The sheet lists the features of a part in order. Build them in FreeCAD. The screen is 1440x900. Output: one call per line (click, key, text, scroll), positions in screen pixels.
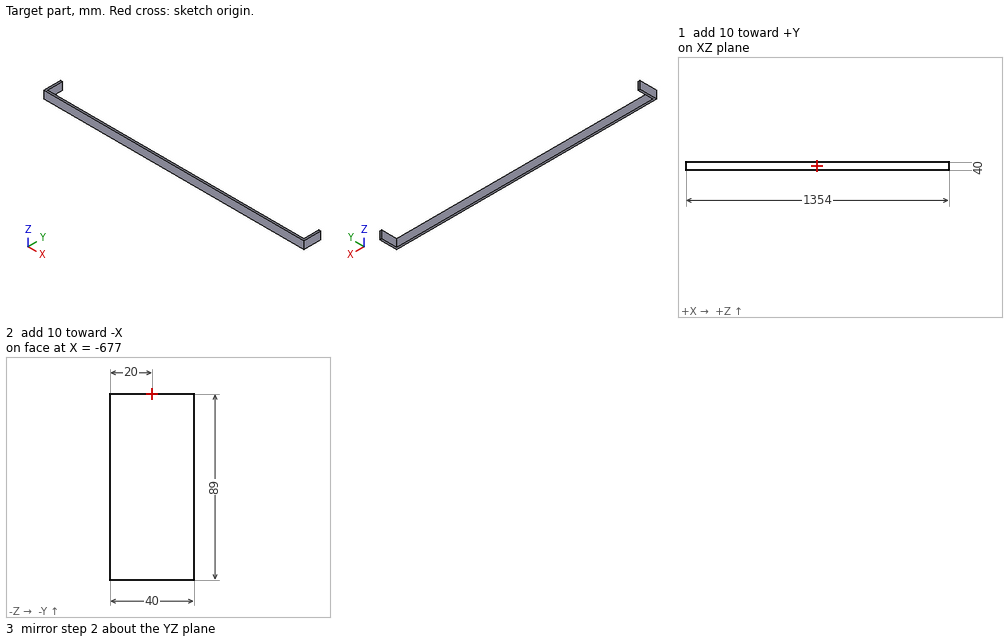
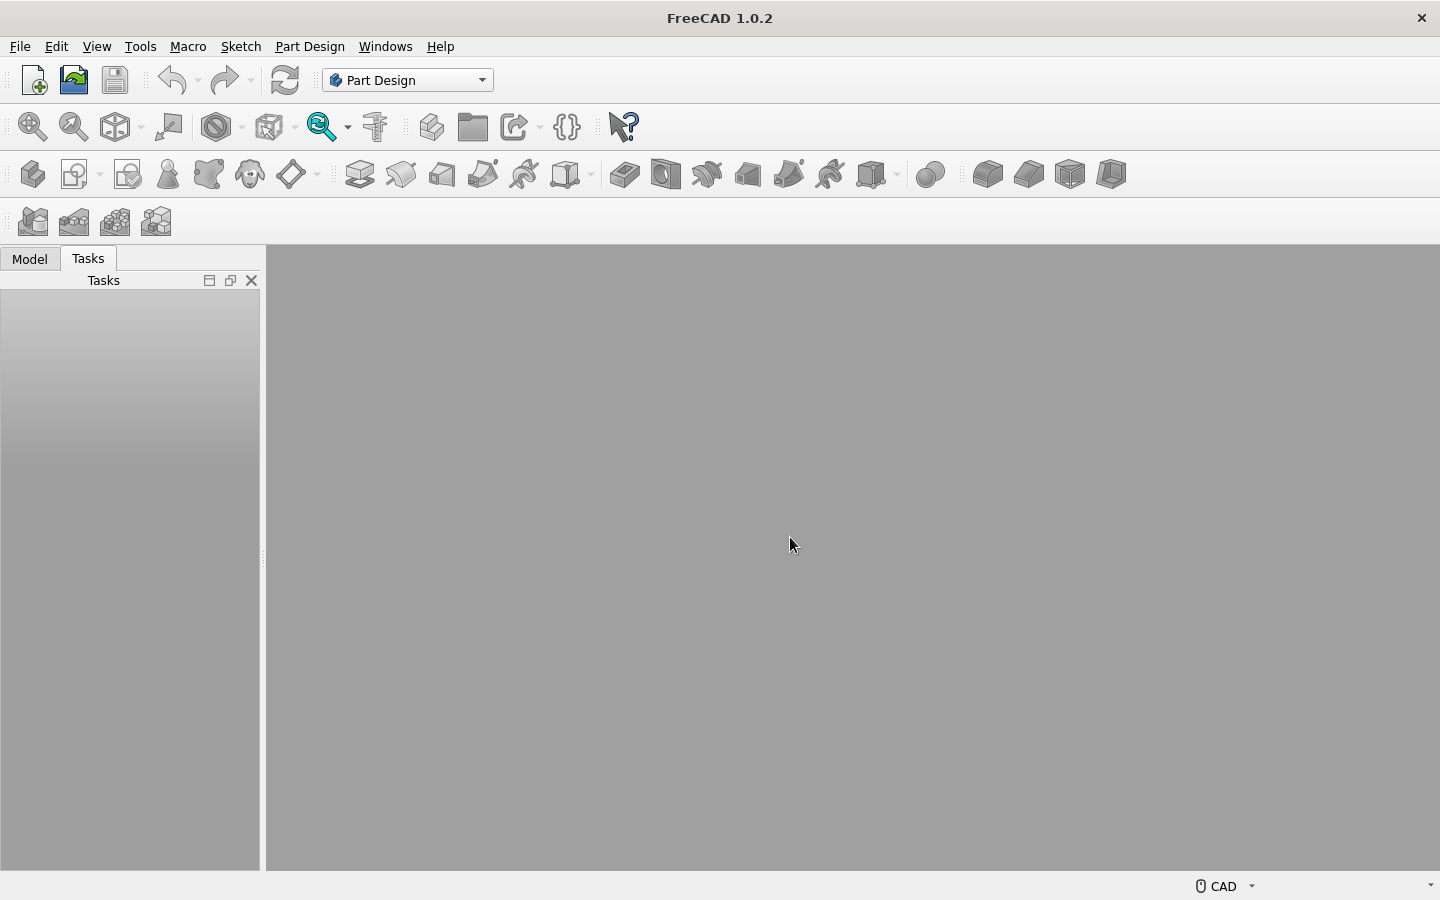
click(33, 80)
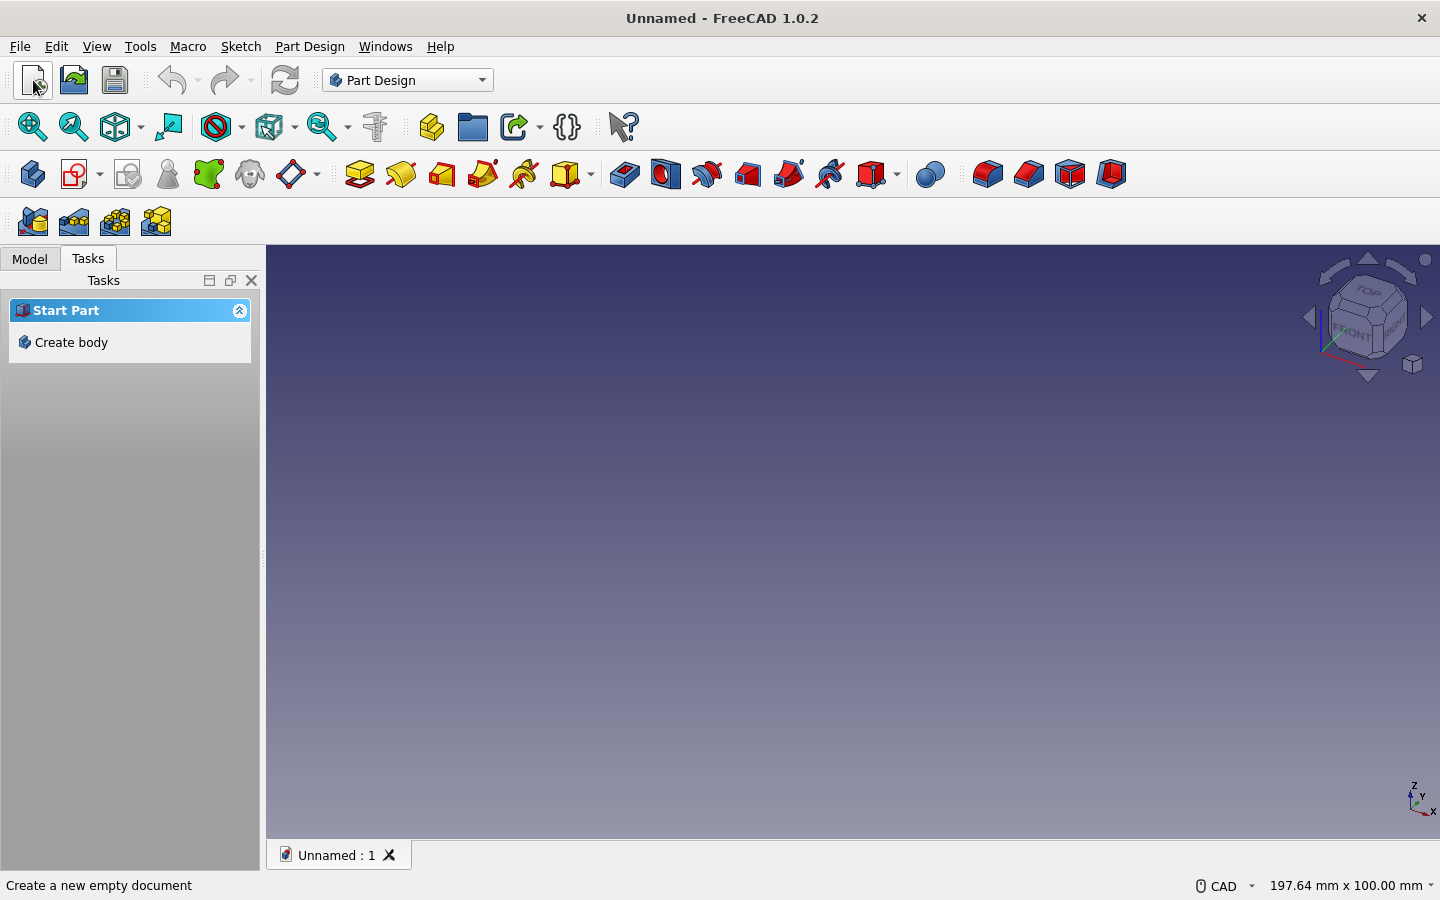
click(74, 174)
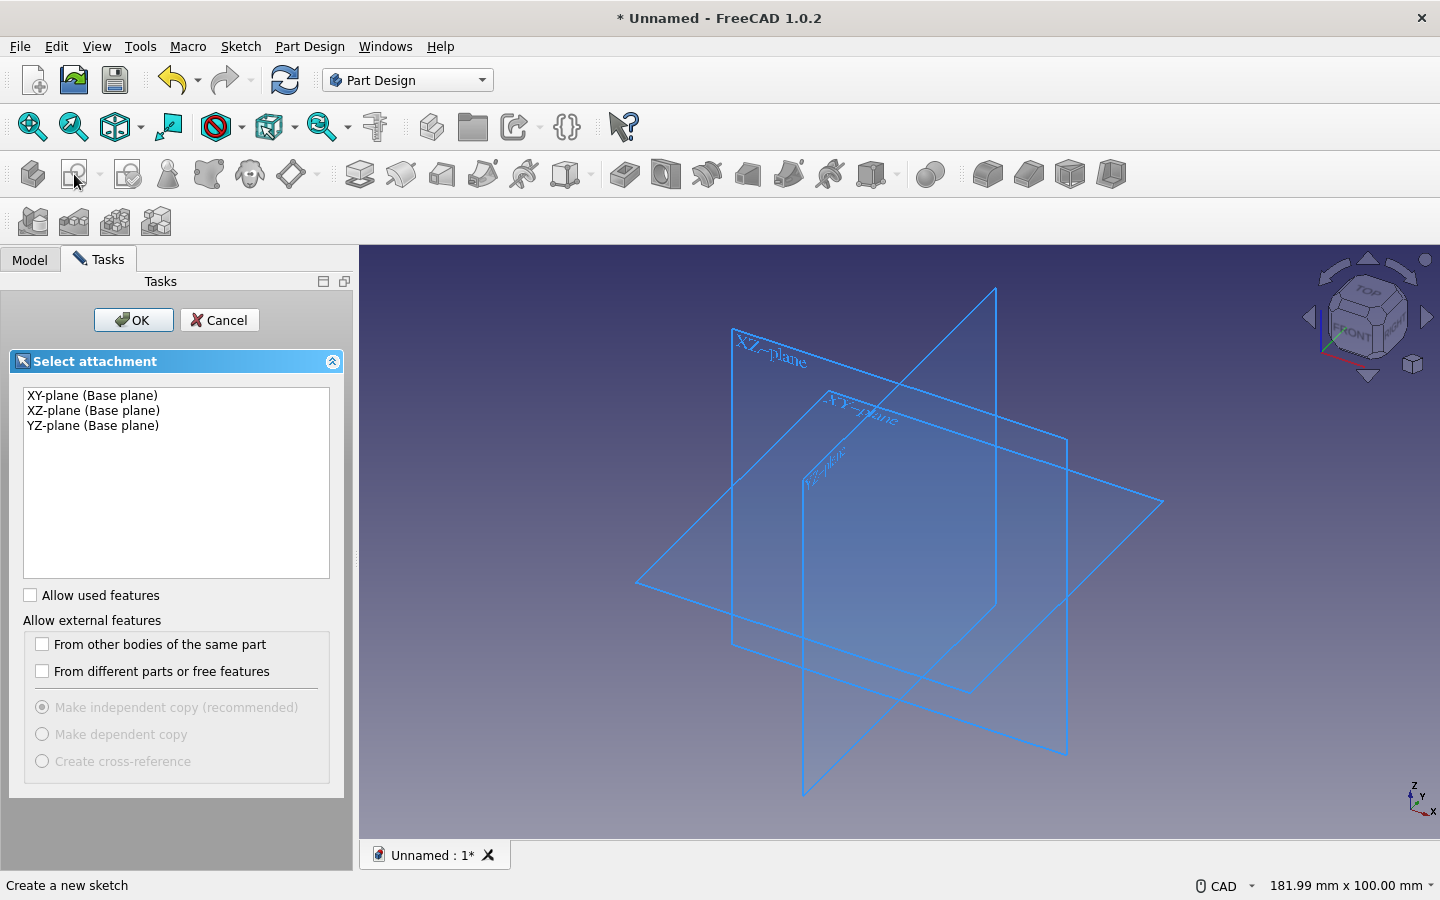
click(84, 410)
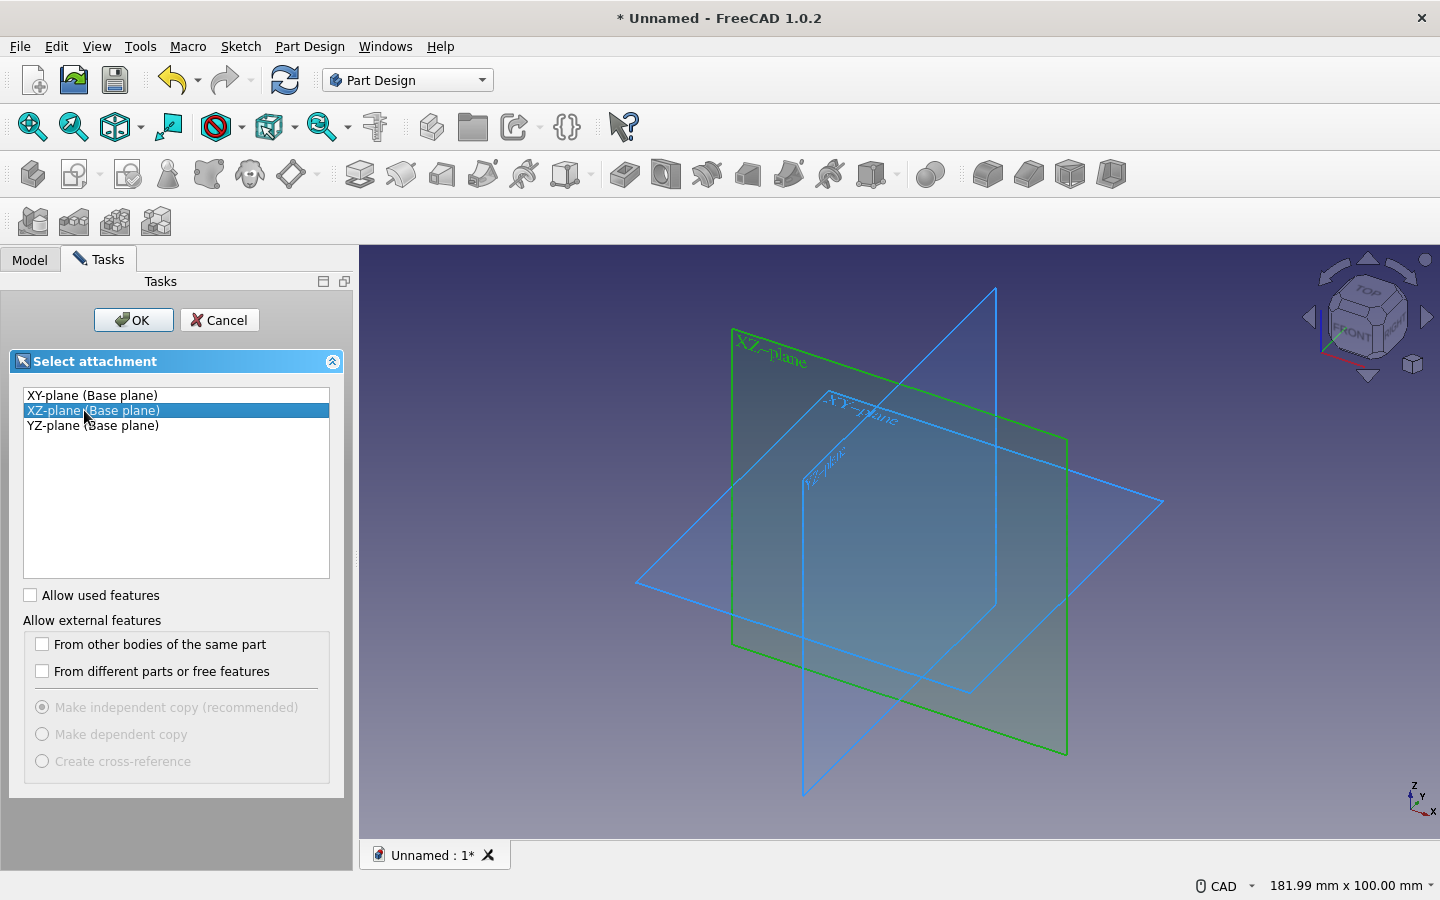
click(134, 320)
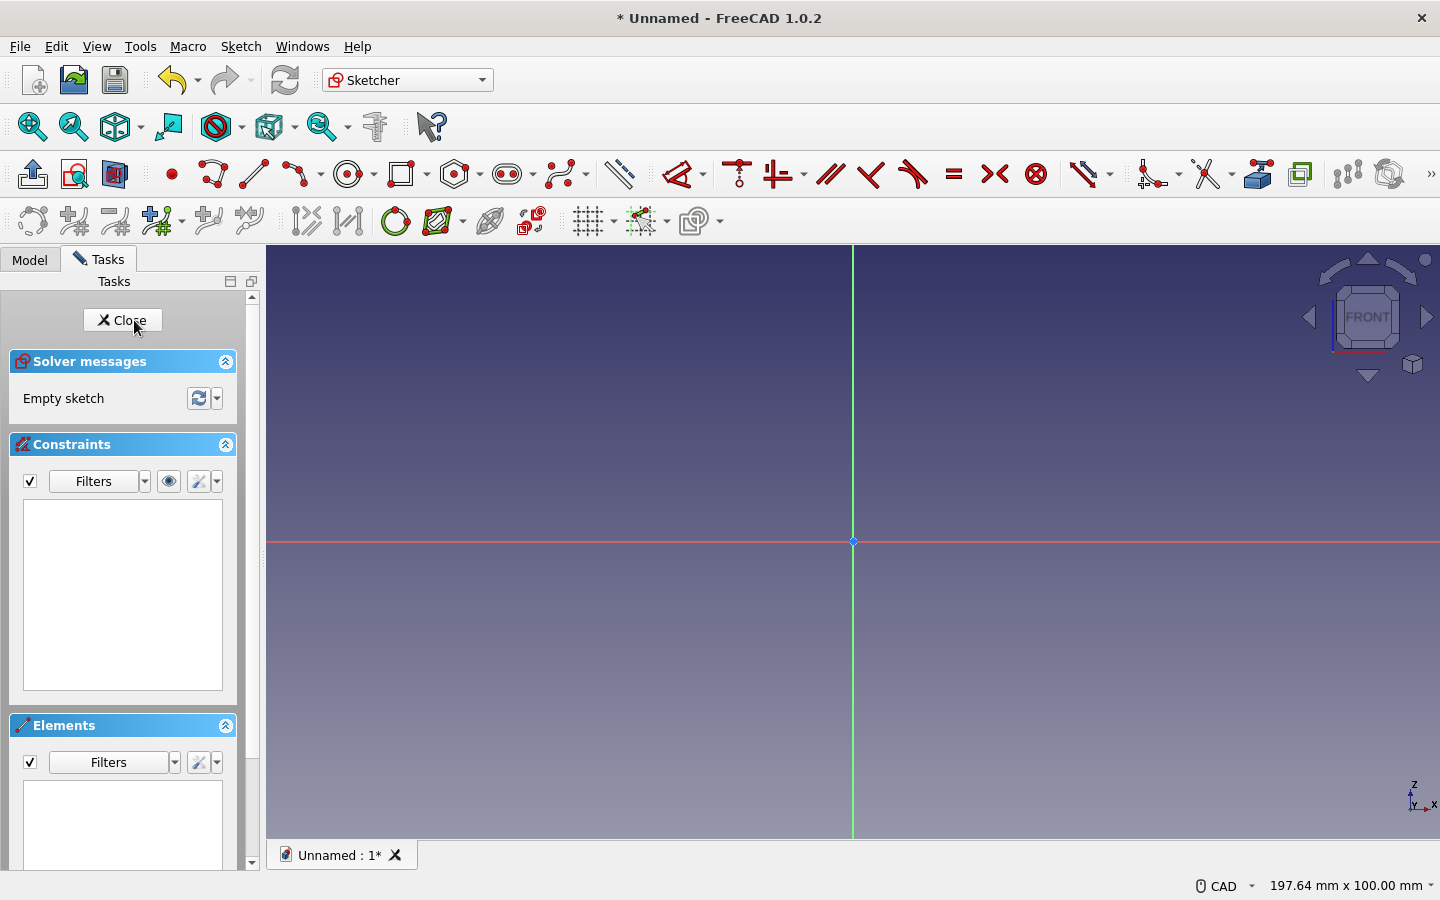
scroll(778, 542, down, 12)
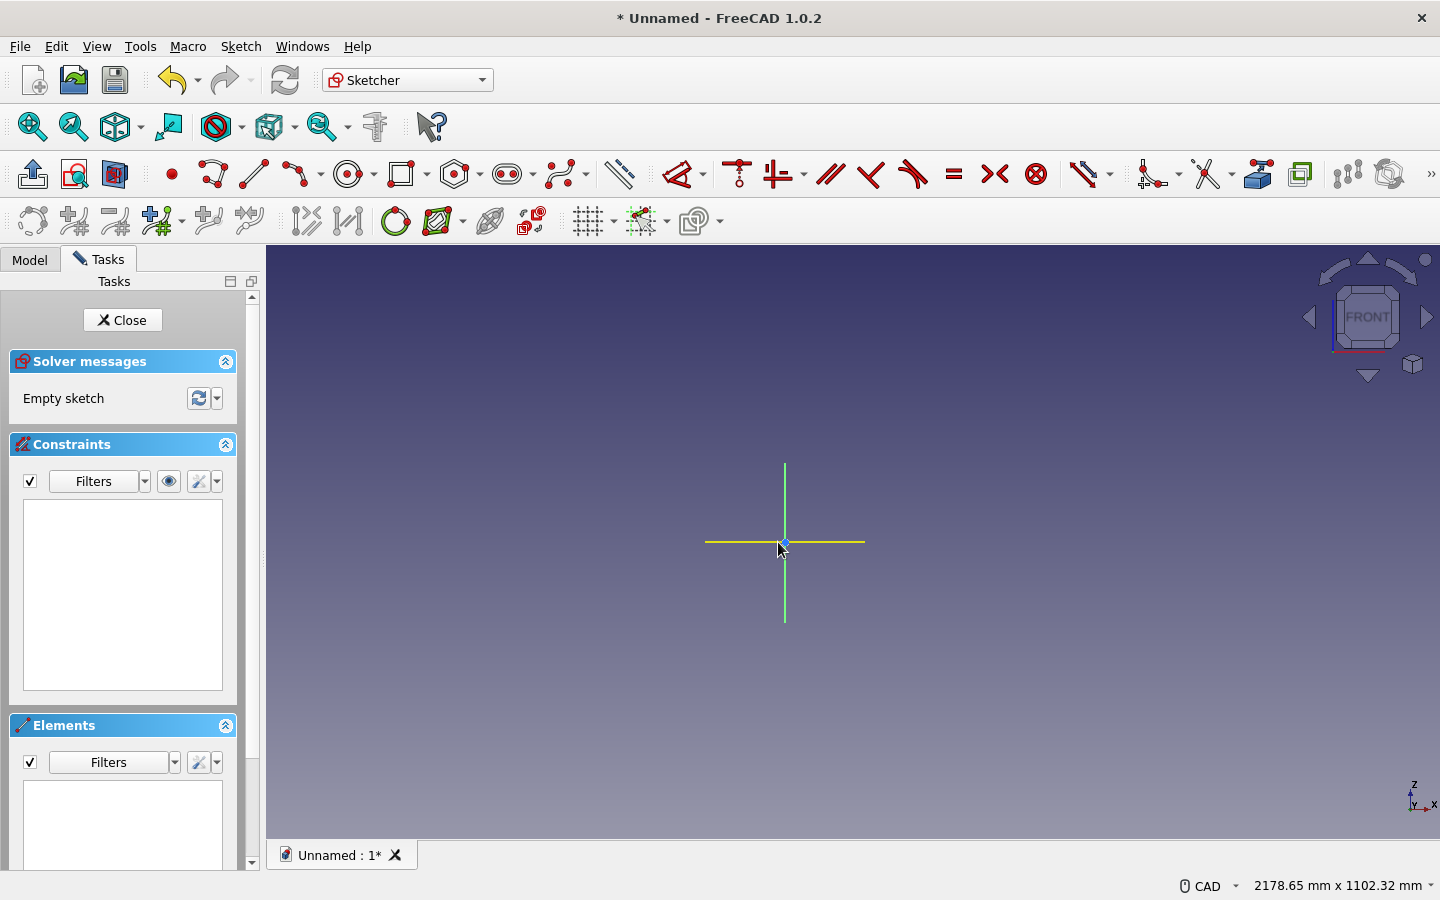
key(g)
key(v)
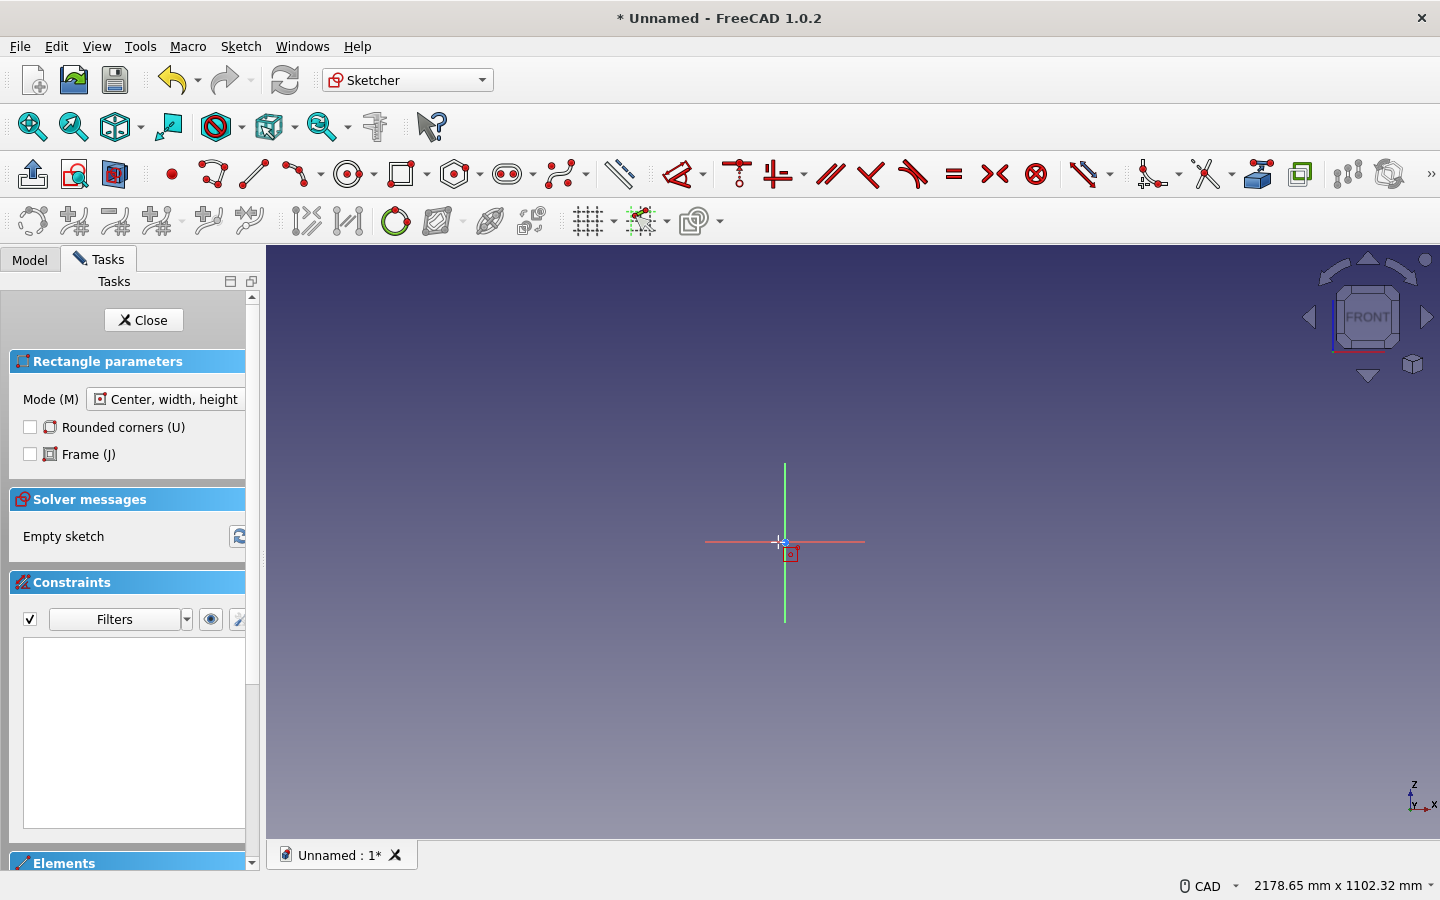
scroll(785, 542, up, 2)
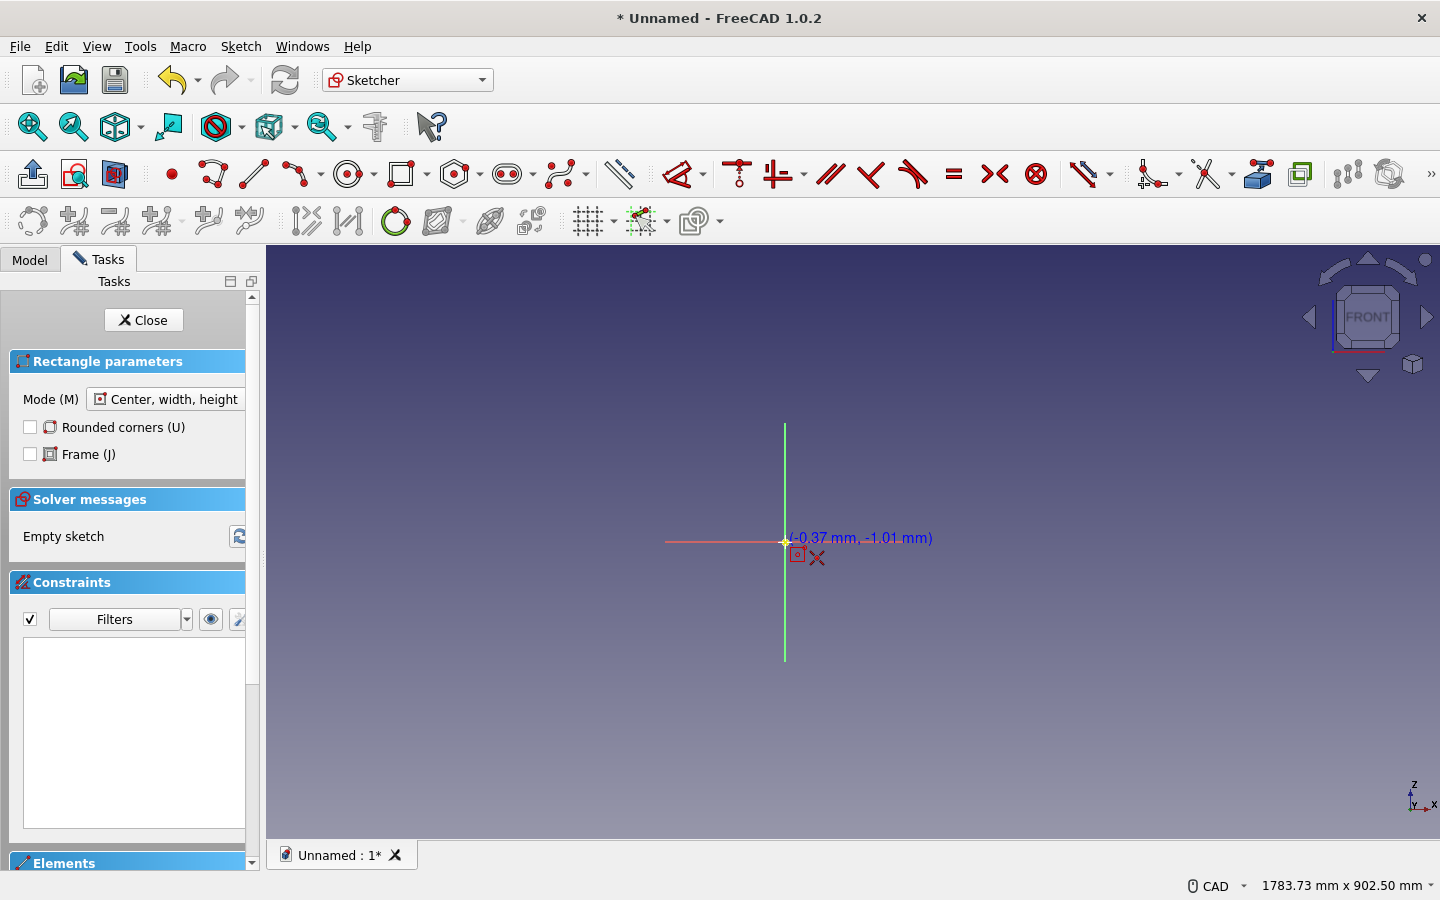
click(785, 542)